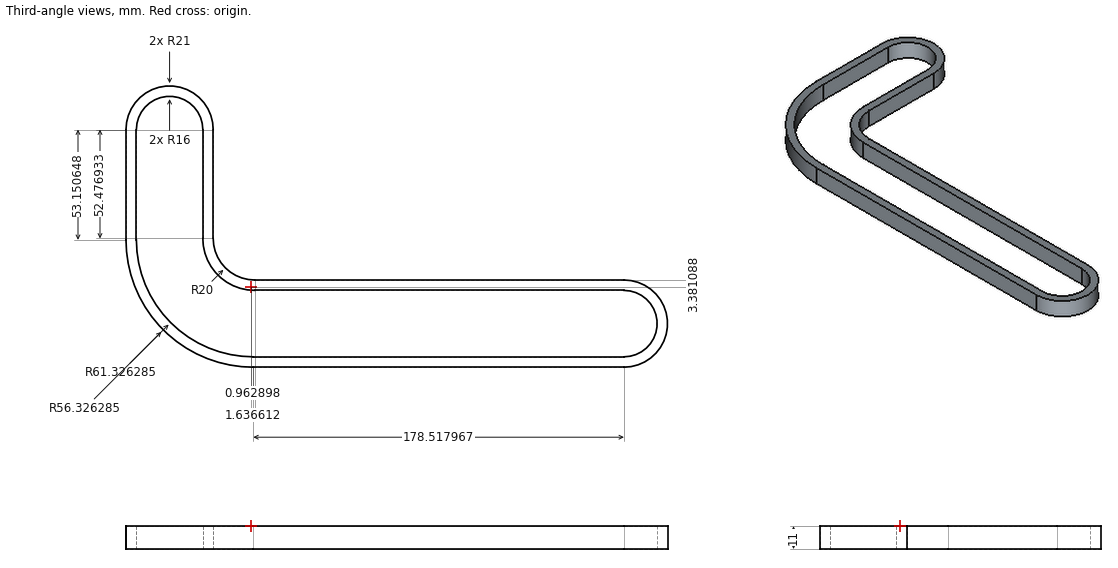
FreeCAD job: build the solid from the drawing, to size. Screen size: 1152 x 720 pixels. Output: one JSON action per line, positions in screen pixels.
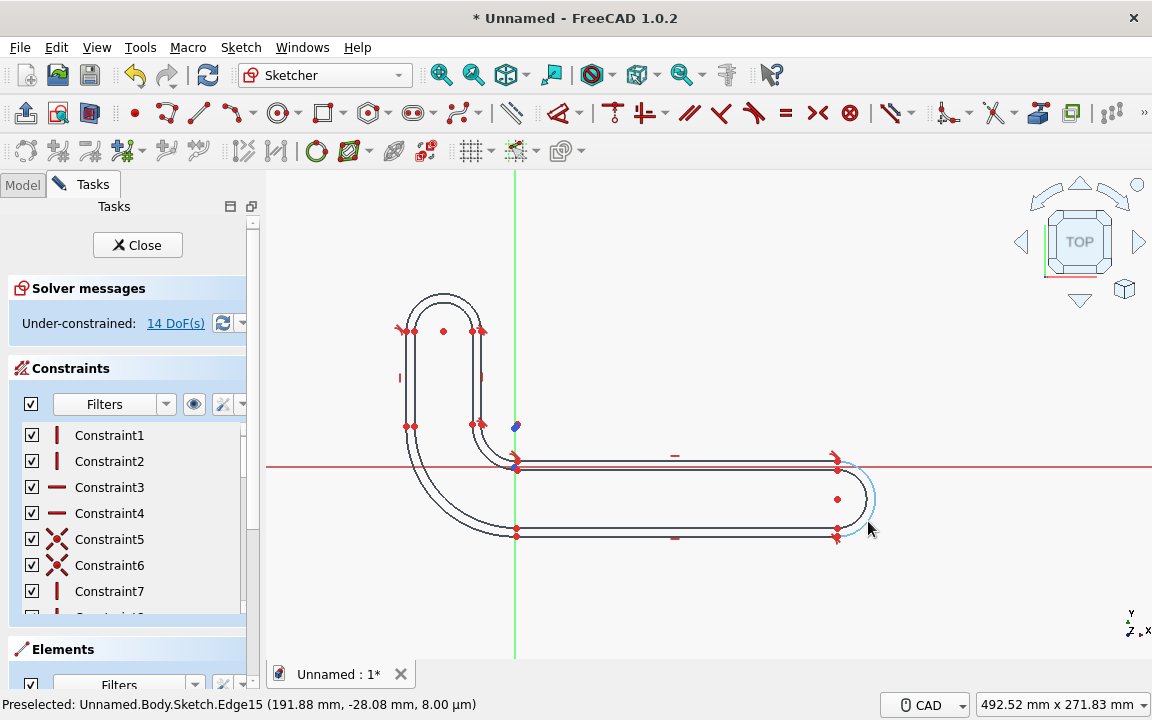
{"action": "scroll", "coordinate": [466, 301], "scroll_direction": "up", "scroll_amount": 3}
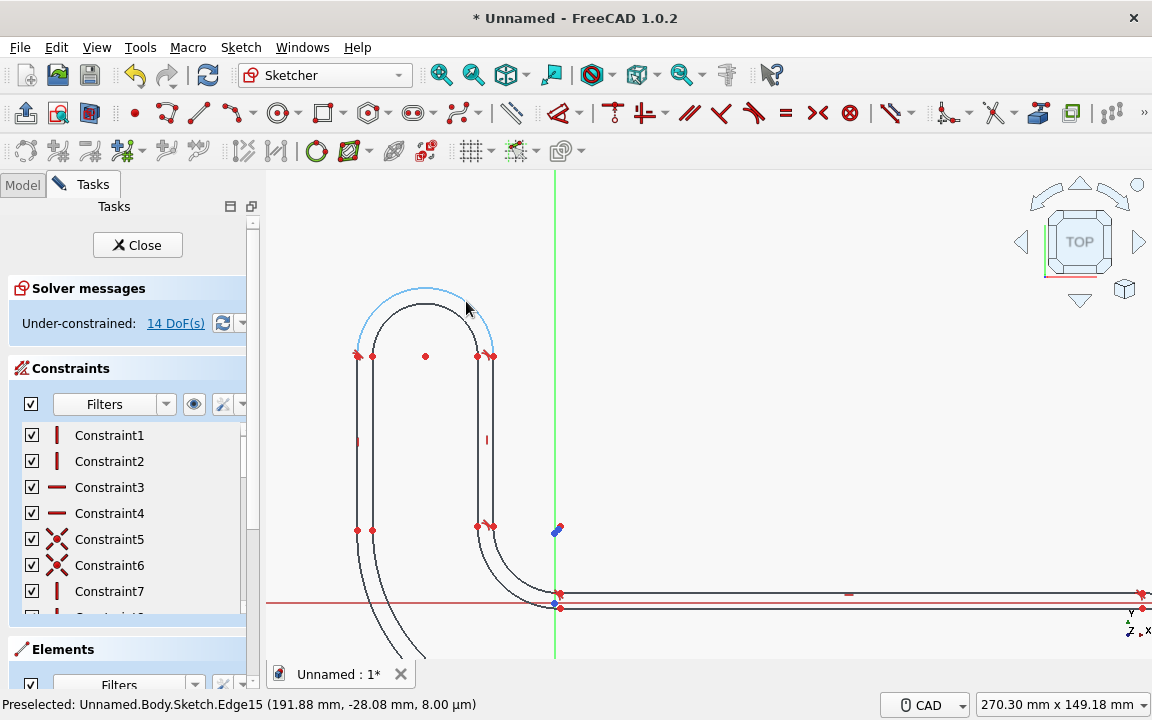
{"action": "left_click", "coordinate": [465, 301]}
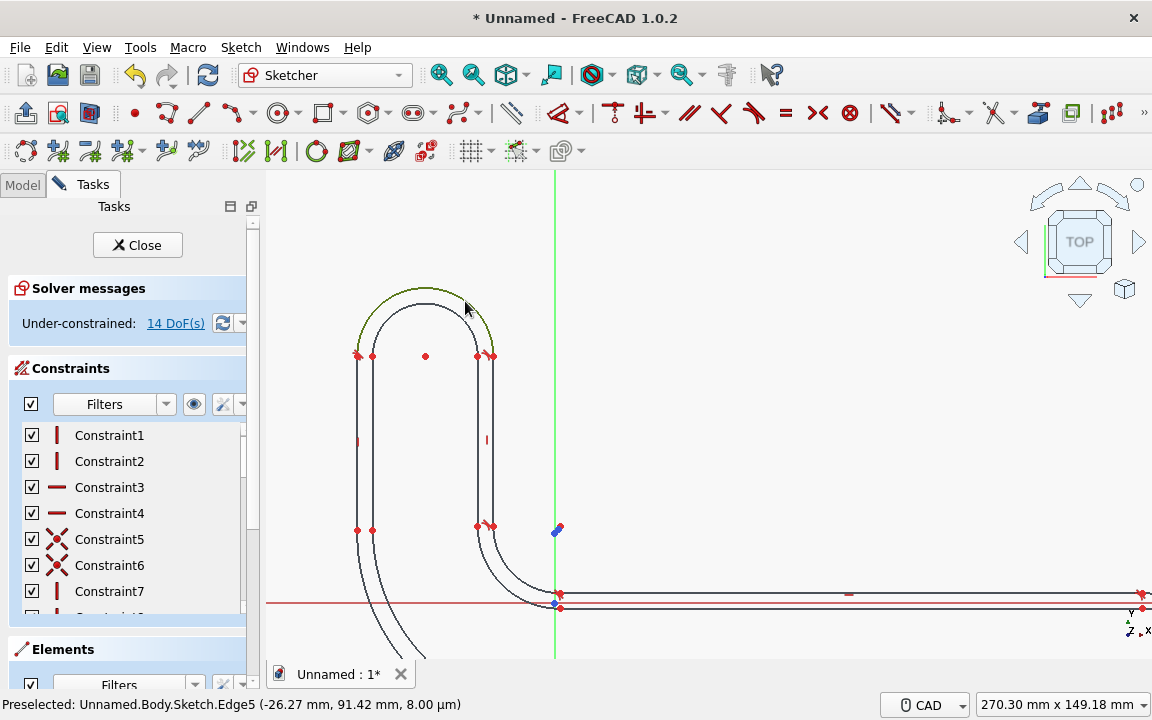
{"action": "scroll", "coordinate": [465, 301], "scroll_direction": "down", "scroll_amount": 3}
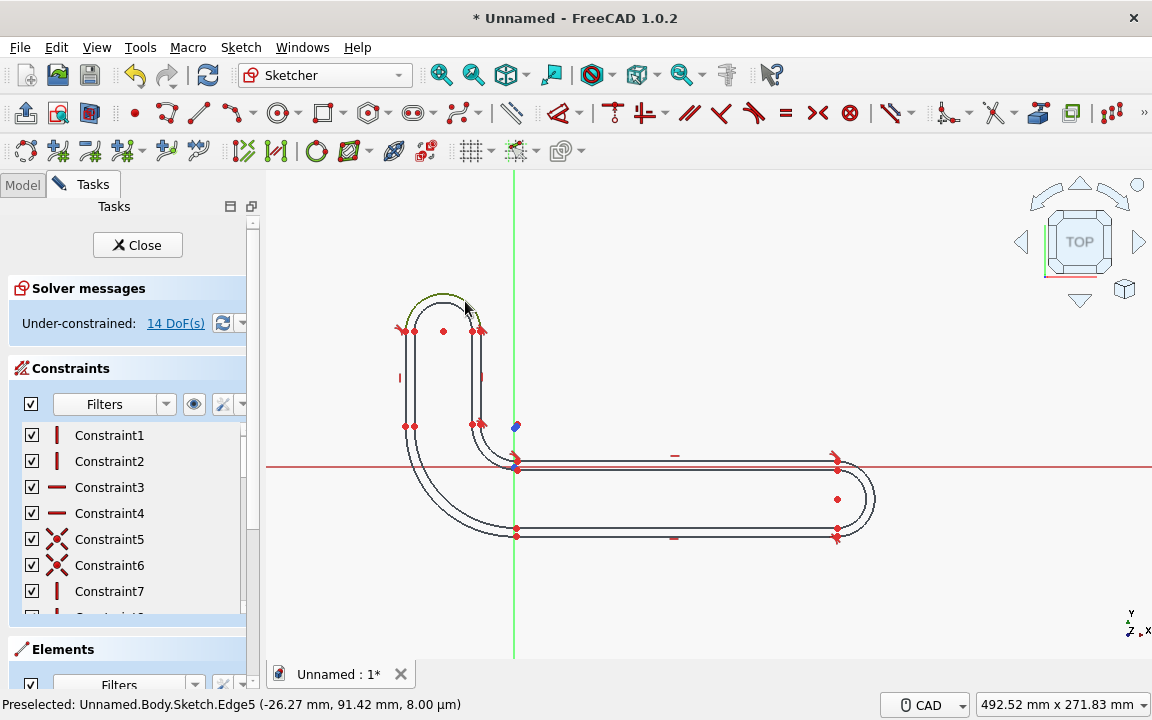
{"action": "scroll", "coordinate": [868, 521], "scroll_direction": "up", "scroll_amount": 3}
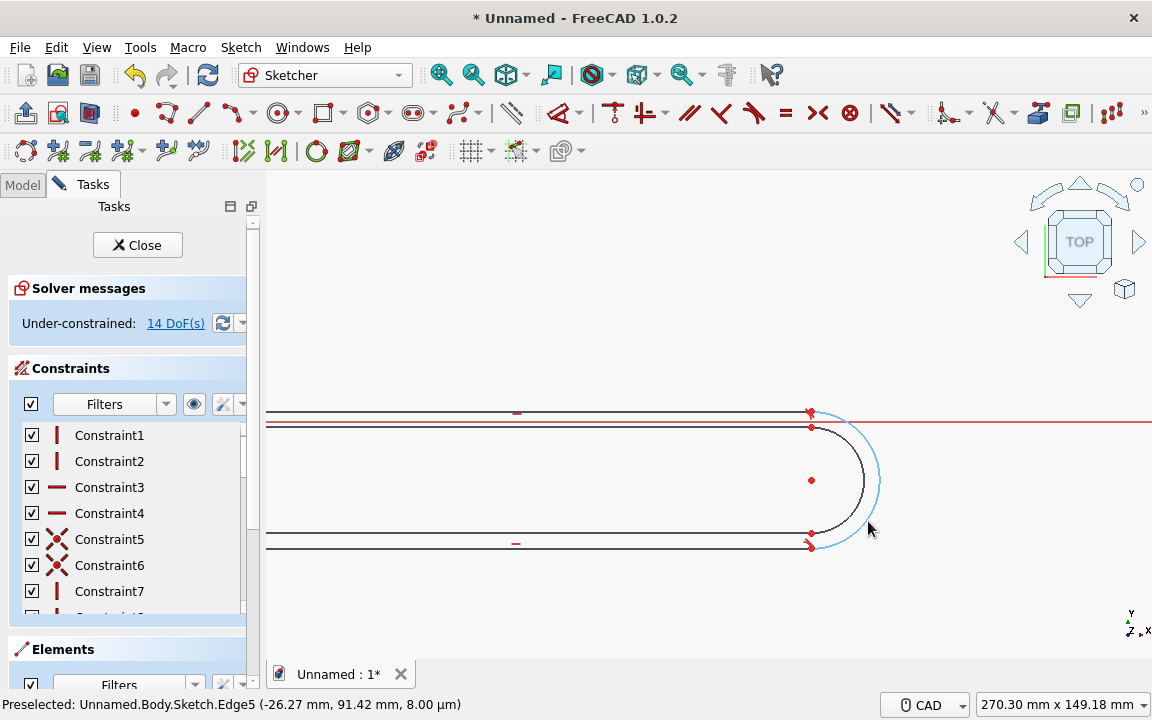
{"action": "left_click", "coordinate": [867, 521]}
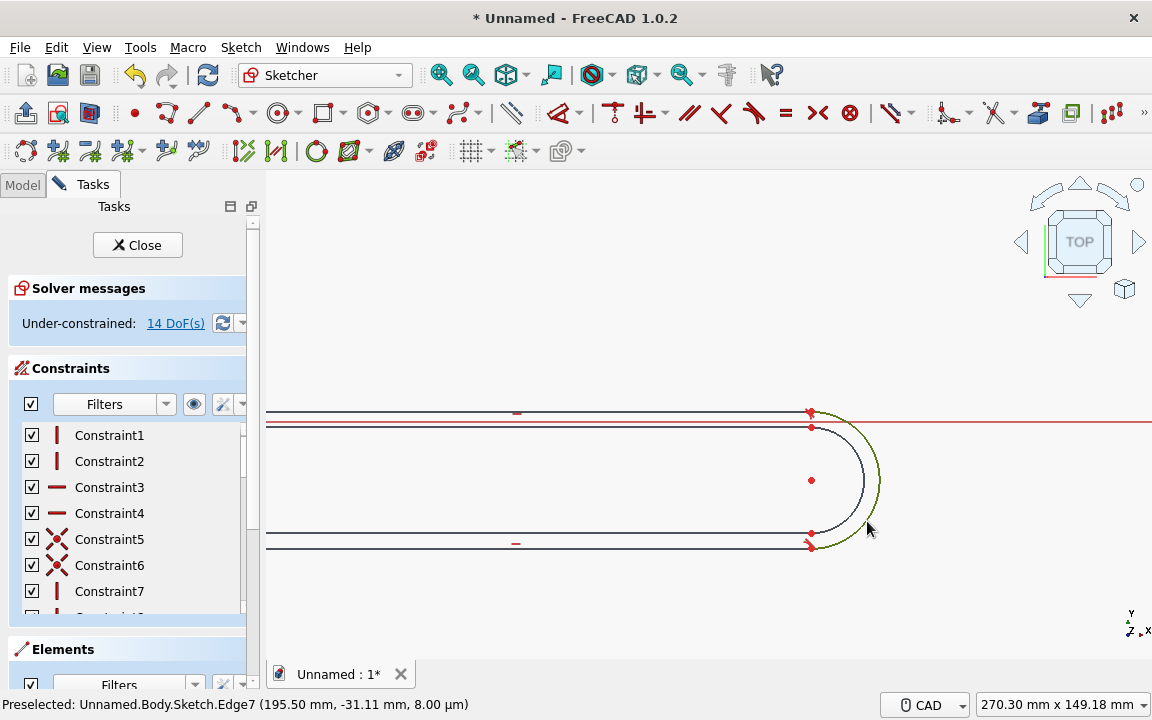
{"action": "left_click", "coordinate": [786, 114]}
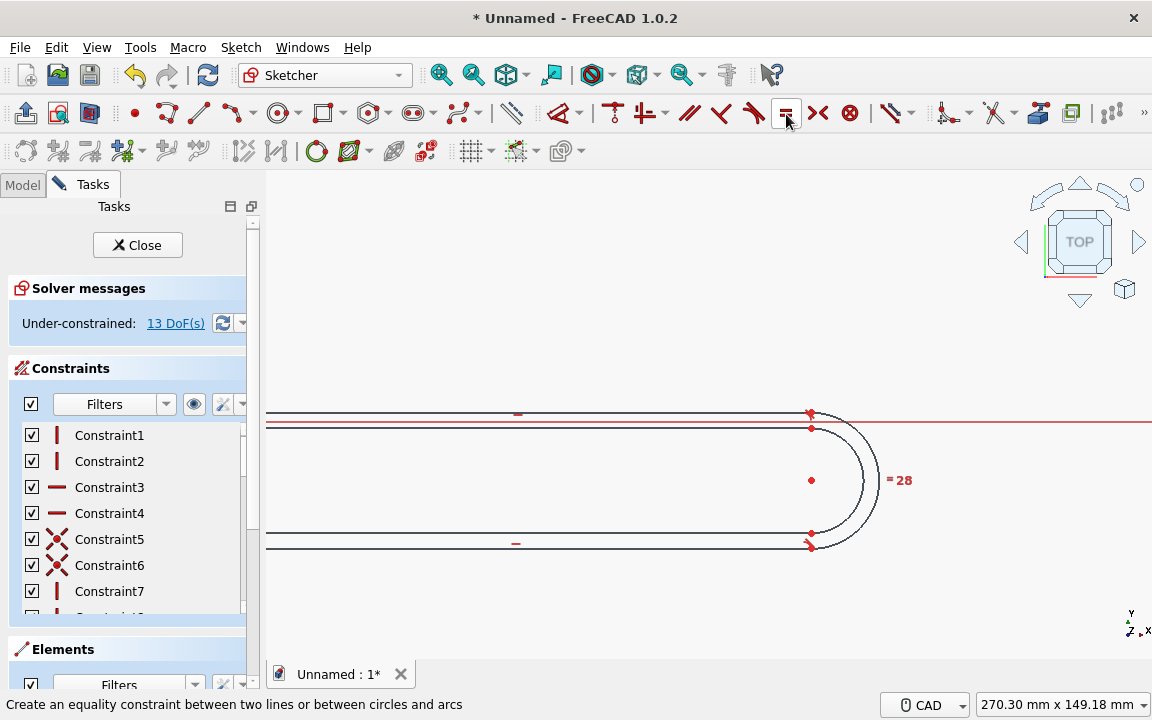
{"action": "left_click", "coordinate": [558, 114]}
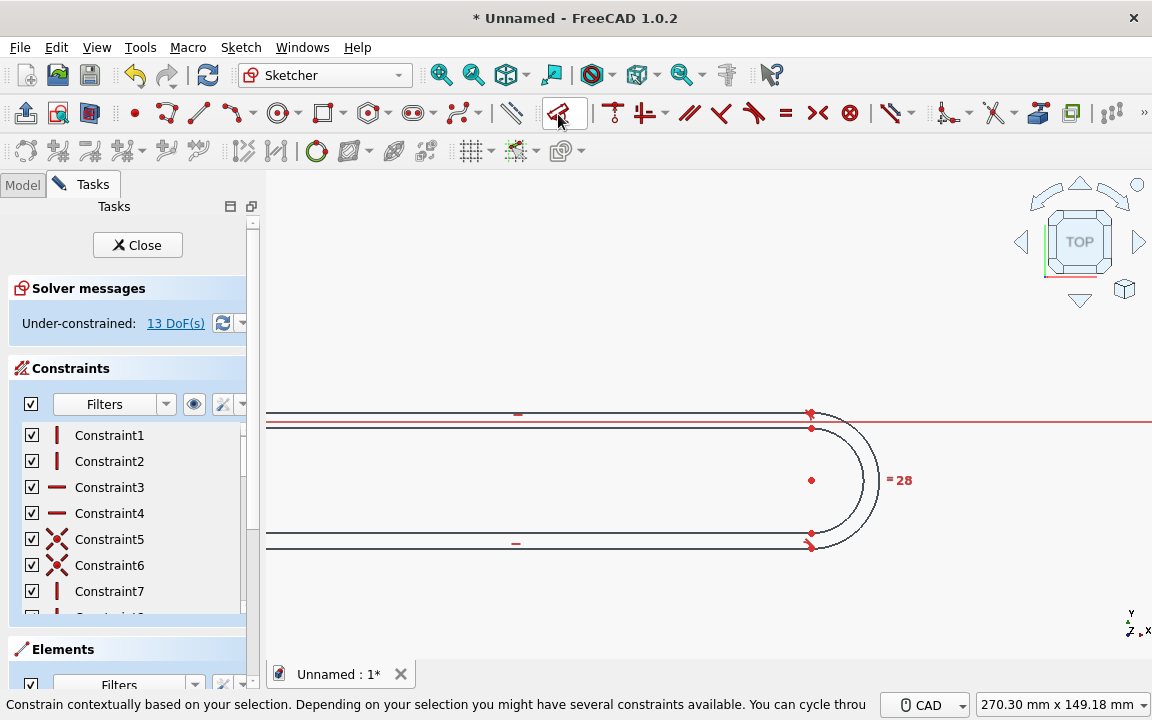
{"action": "scroll", "coordinate": [869, 521], "scroll_direction": "down", "scroll_amount": 3}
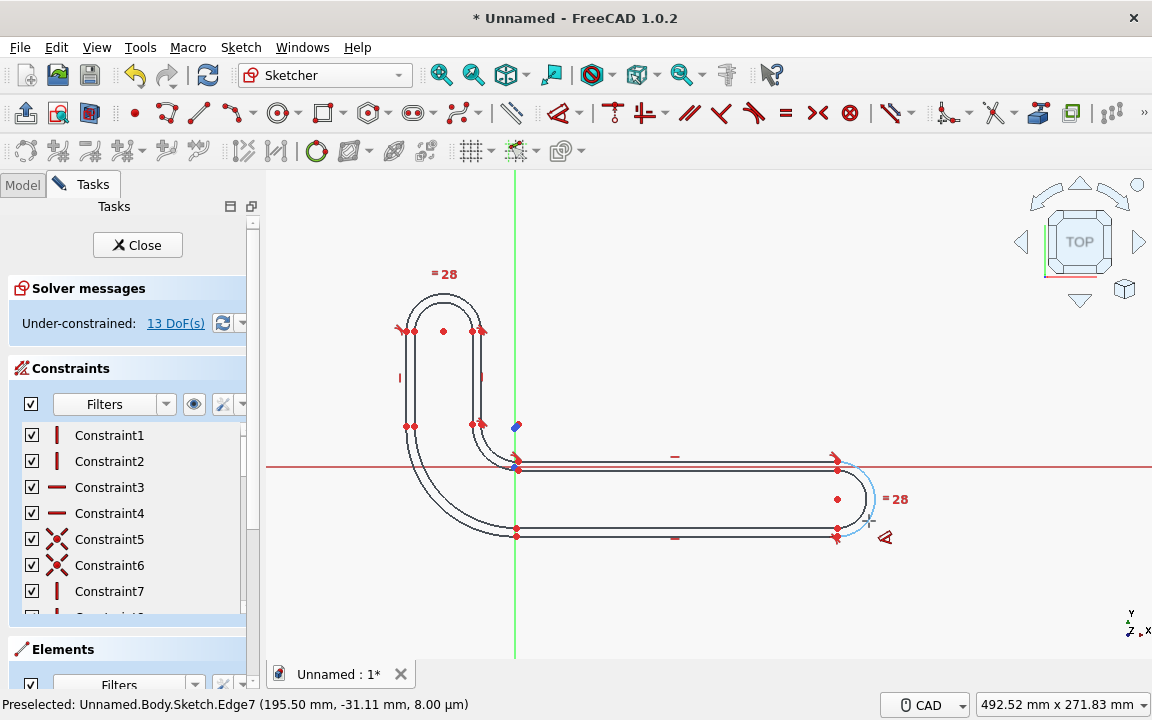
{"action": "scroll", "coordinate": [466, 301], "scroll_direction": "up", "scroll_amount": 3}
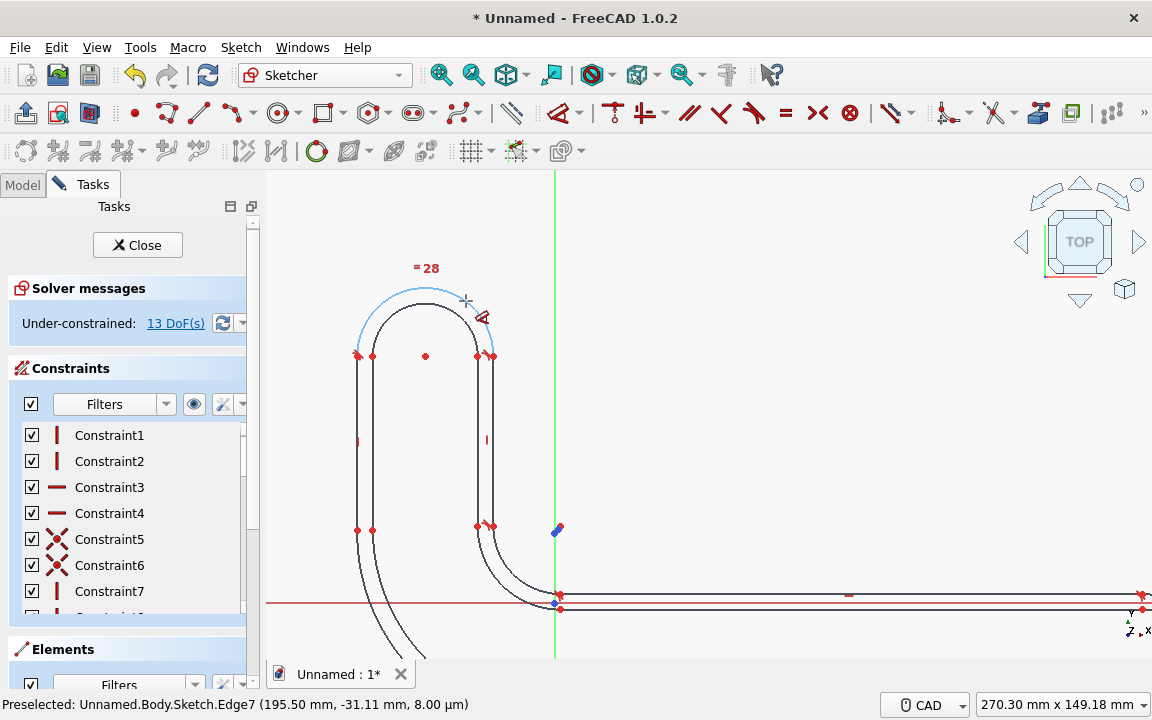
{"action": "left_click", "coordinate": [465, 301]}
{"action": "left_click", "coordinate": [484, 275]}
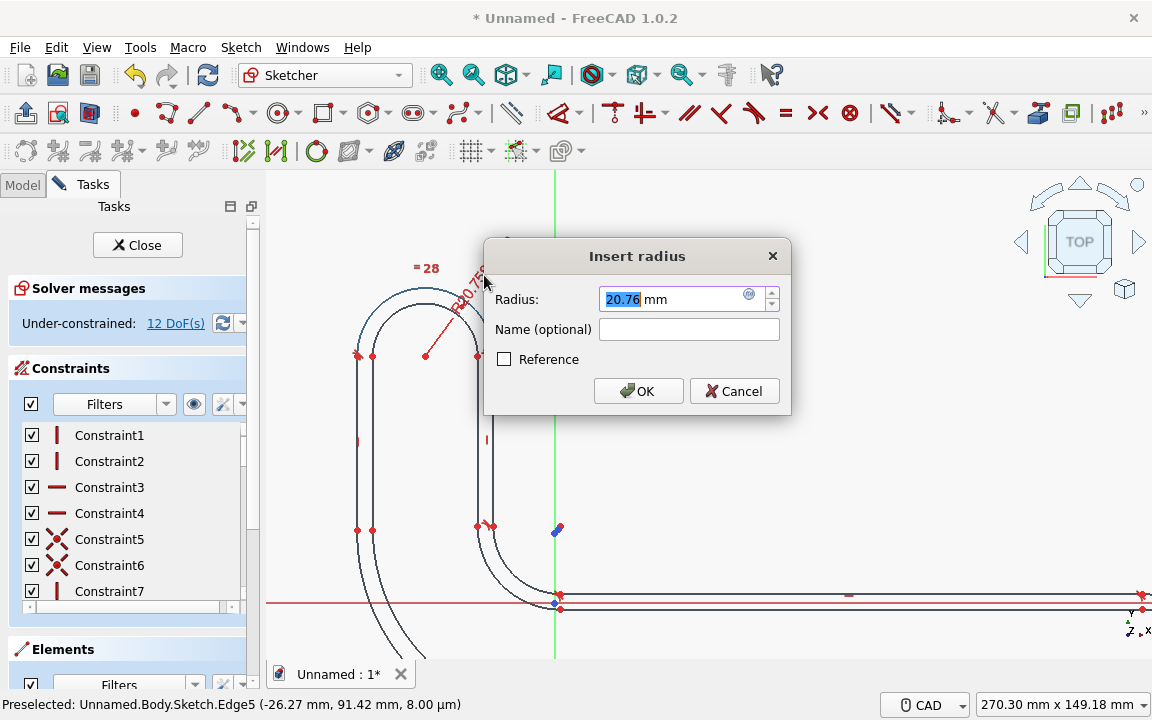
{"action": "type", "text": "21"}
{"action": "key", "text": "Return"}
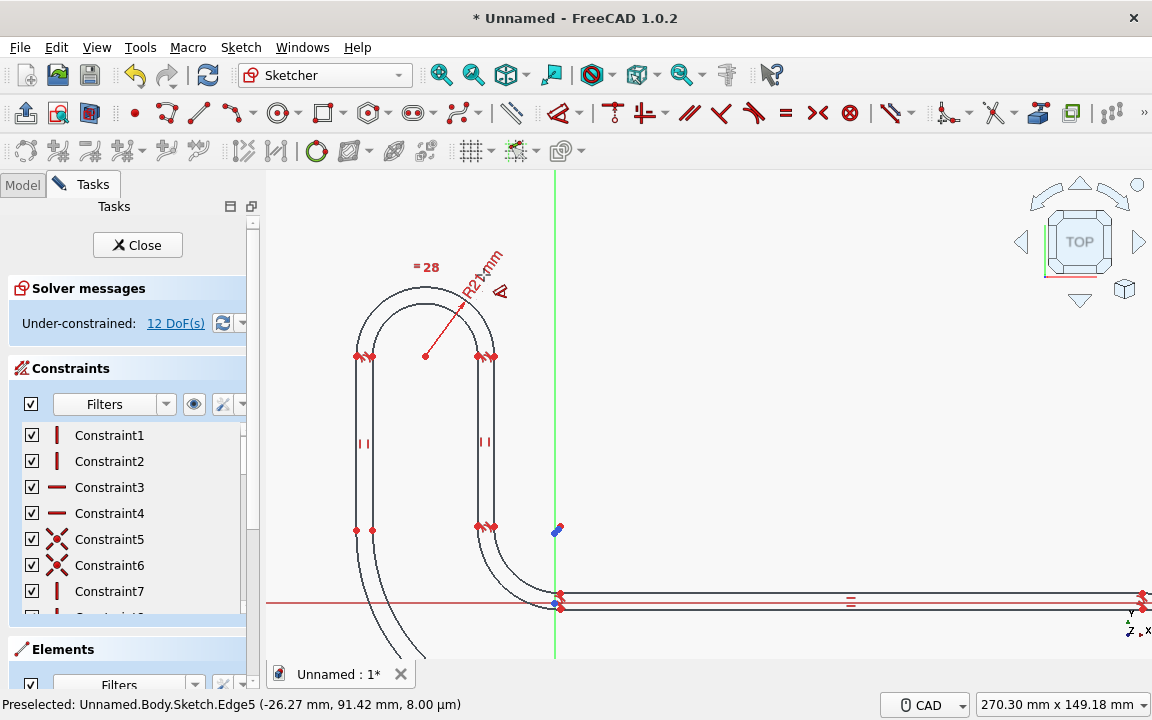
{"action": "left_click", "coordinate": [378, 622]}
{"action": "left_click", "coordinate": [325, 526]}